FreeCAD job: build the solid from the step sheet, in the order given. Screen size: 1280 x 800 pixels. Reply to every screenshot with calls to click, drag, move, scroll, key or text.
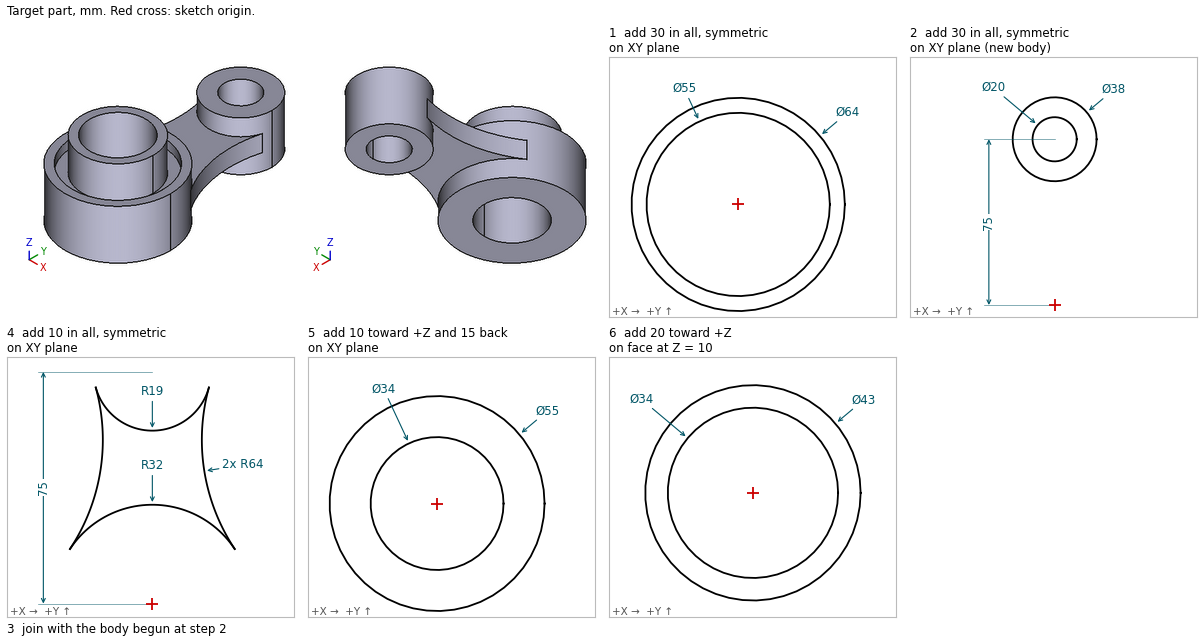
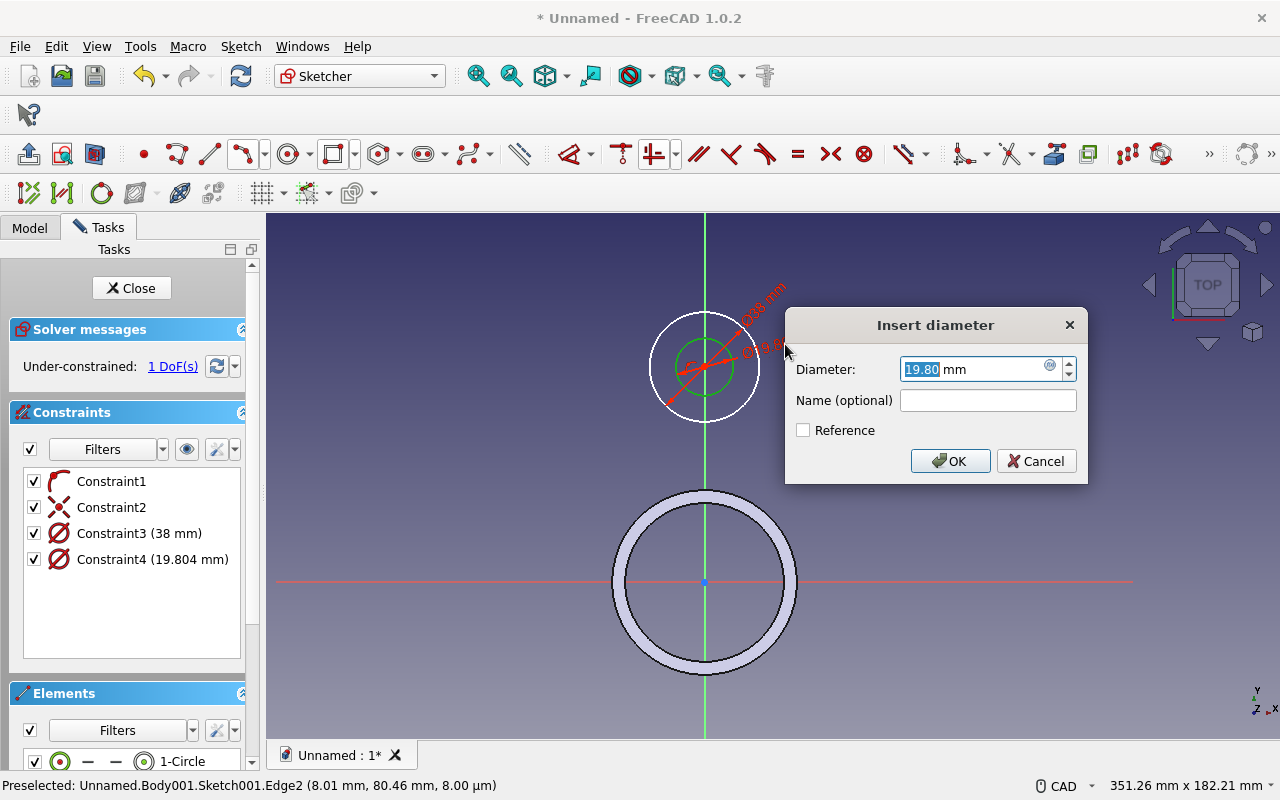
text(20)
key(Return)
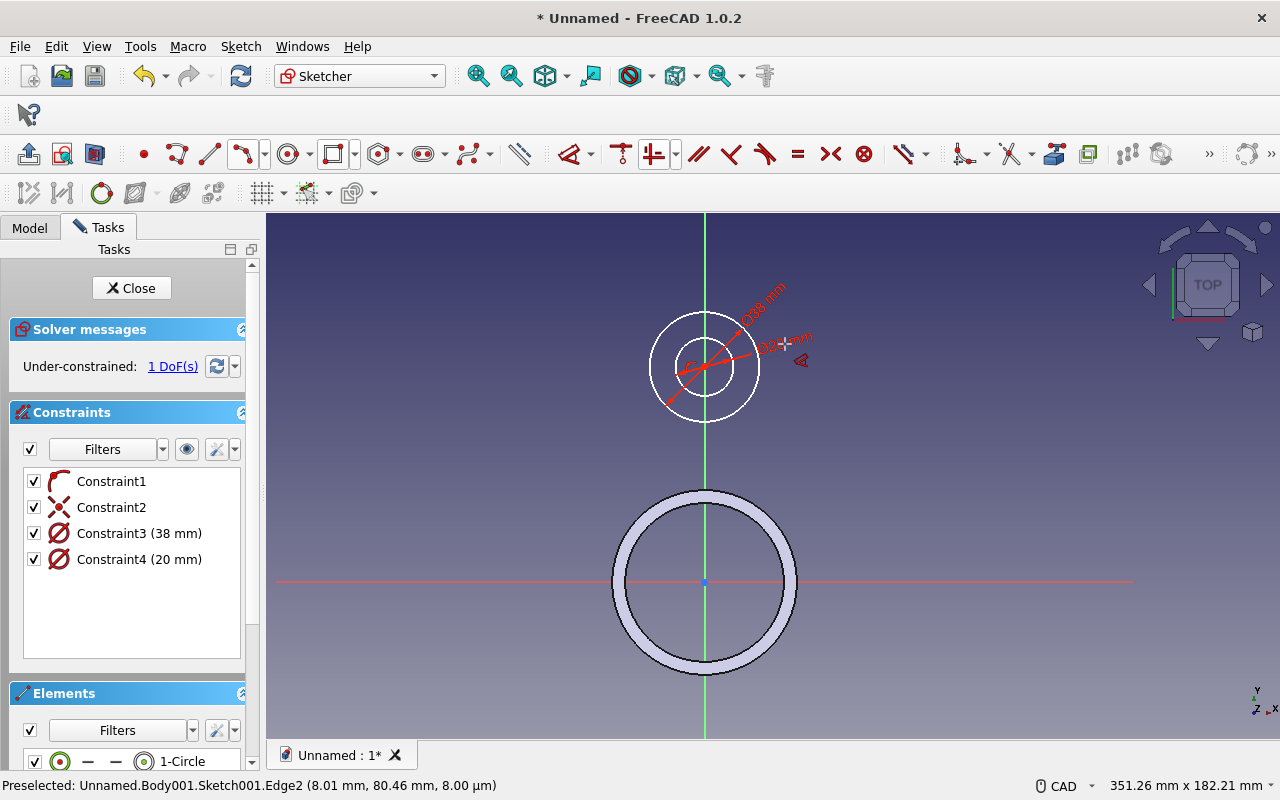
click(705, 367)
click(739, 475)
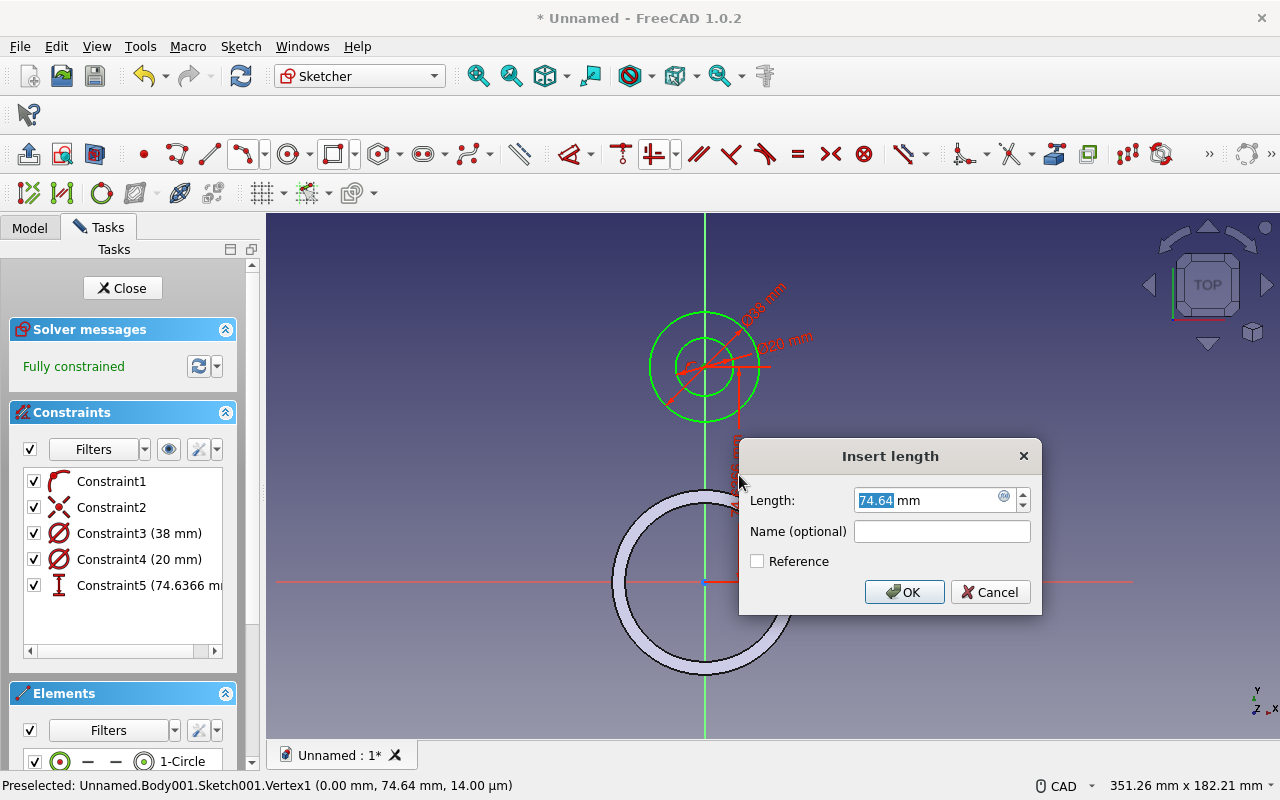
text(75)
key(Return)
key(Escape)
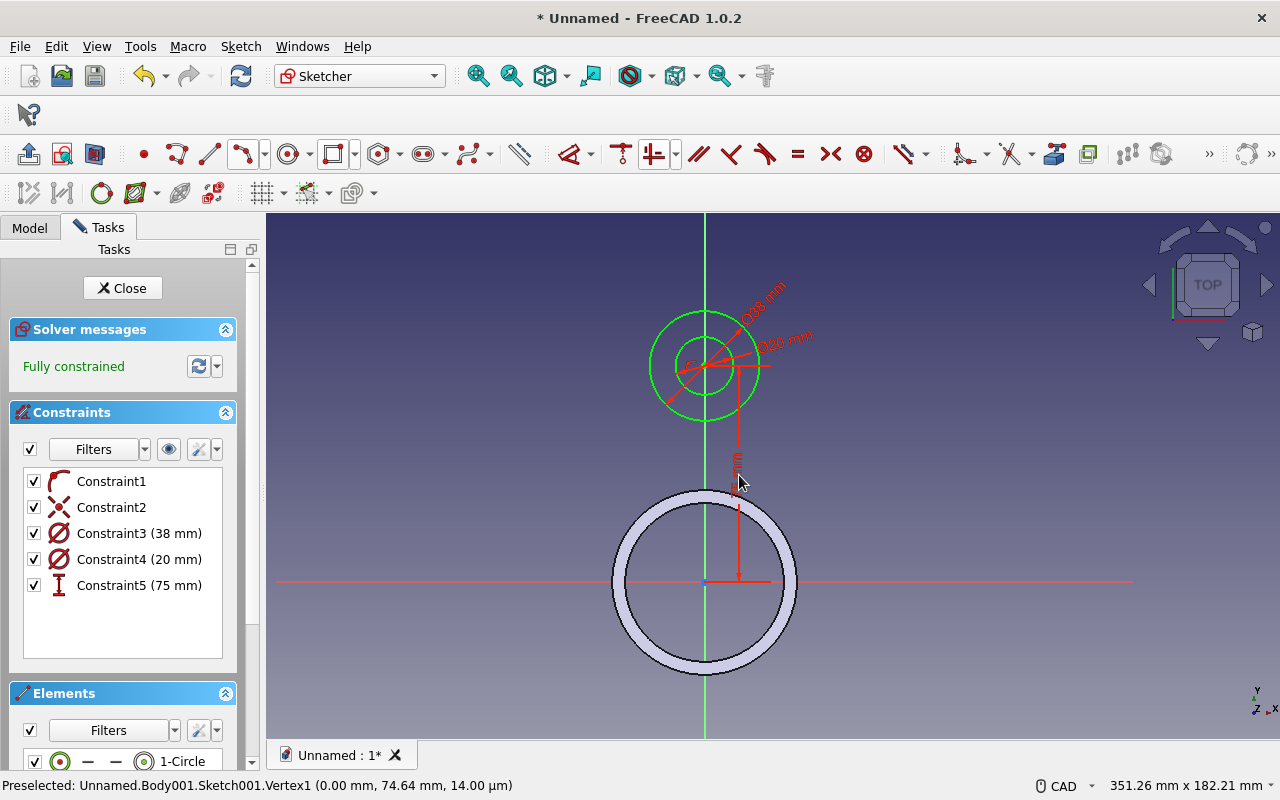
click(123, 288)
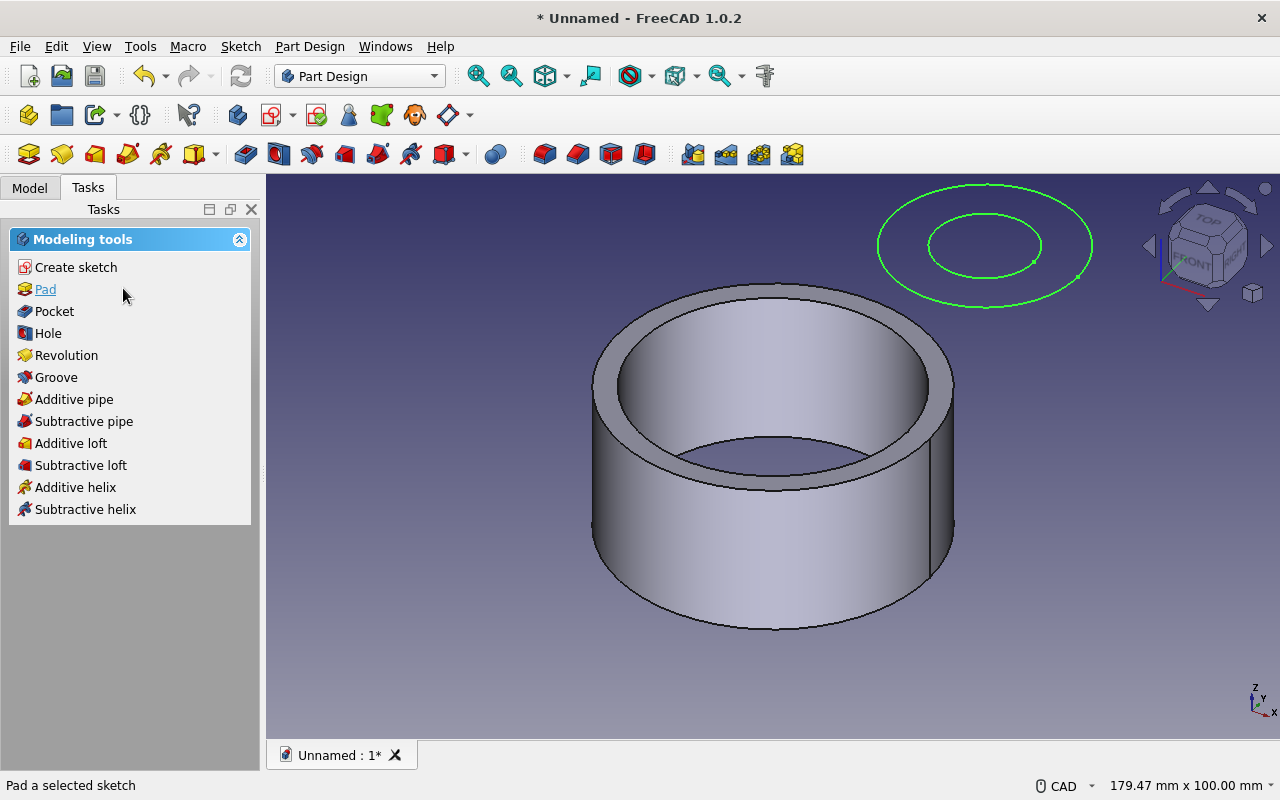
click(29, 154)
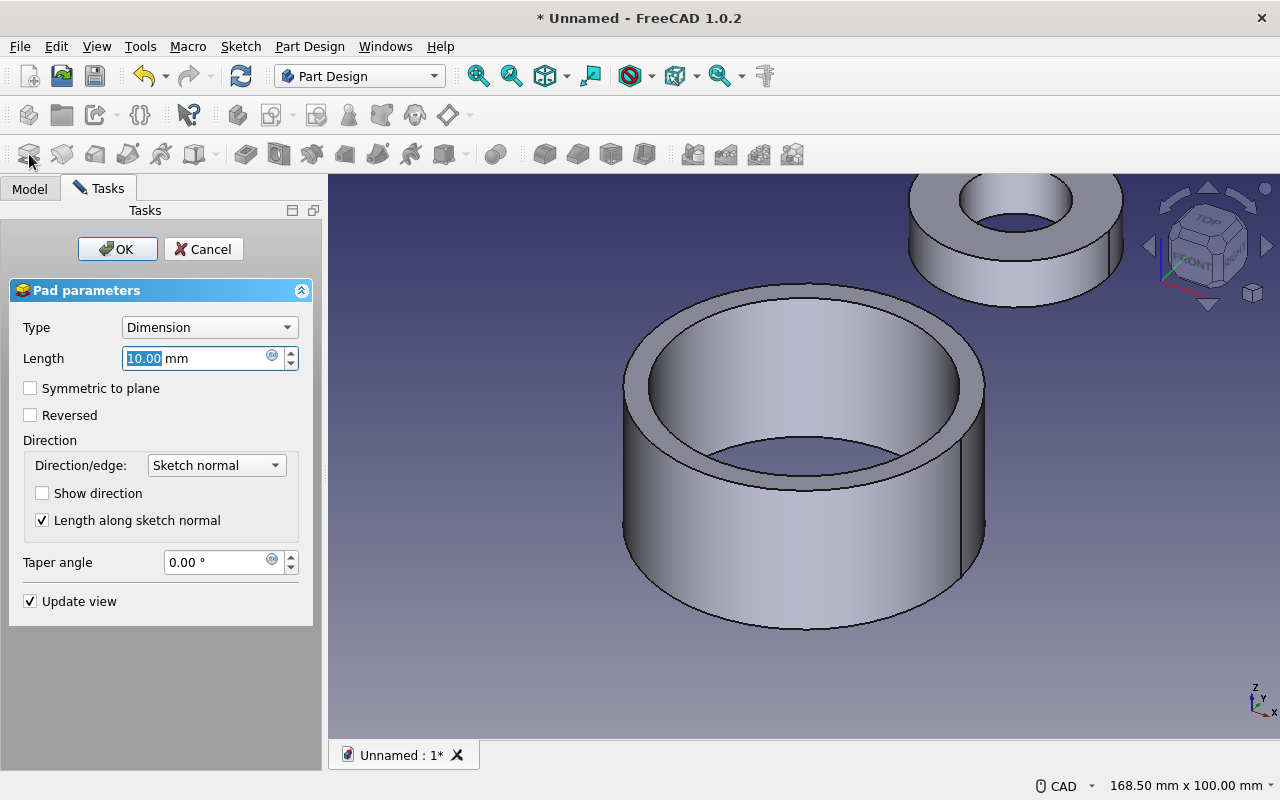
text(30)
key(Tab)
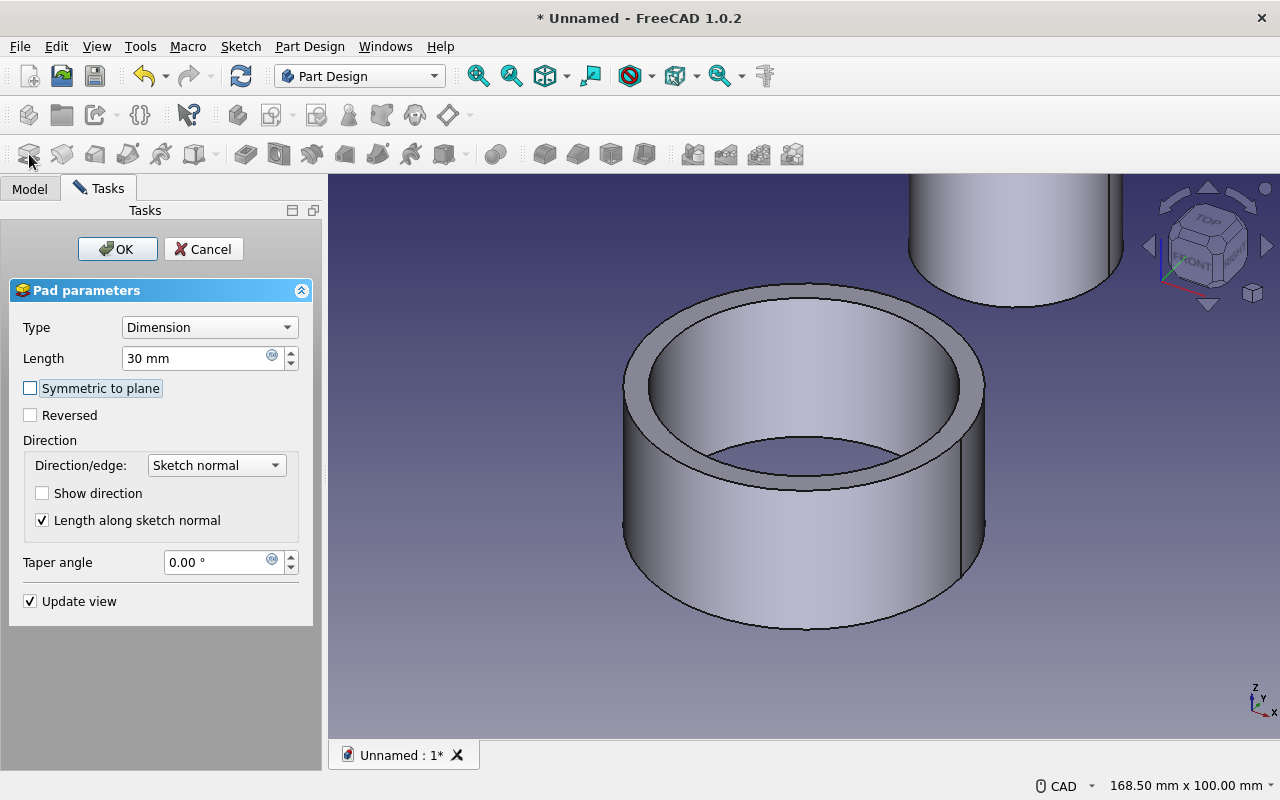
click(31, 388)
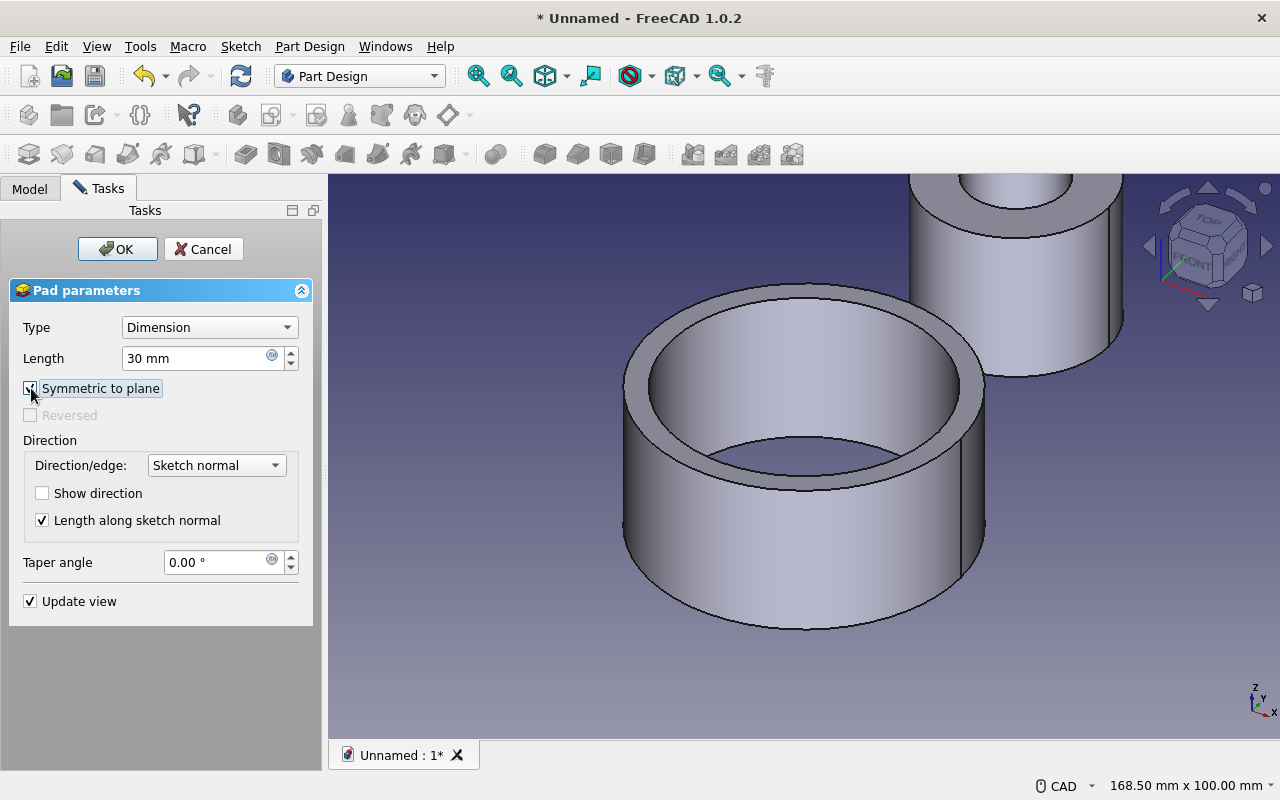
click(118, 249)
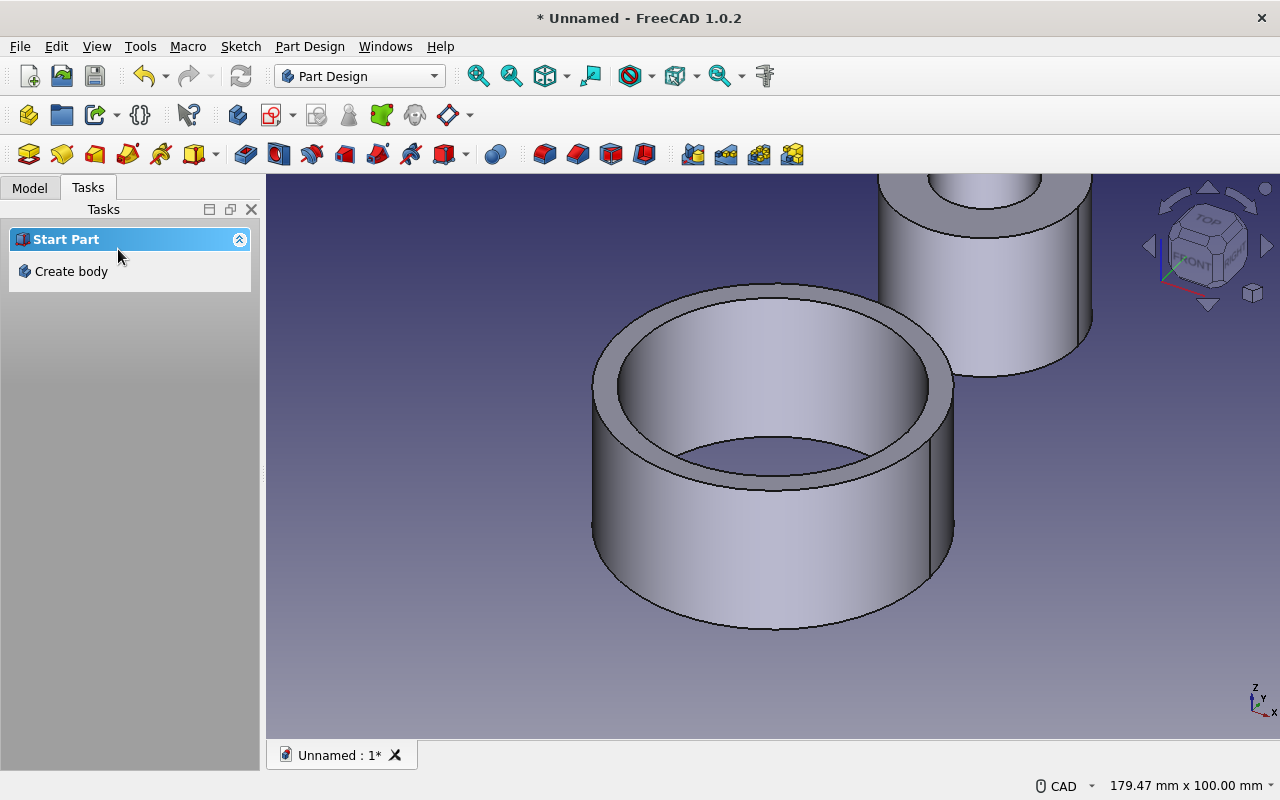
key(v)
key(f)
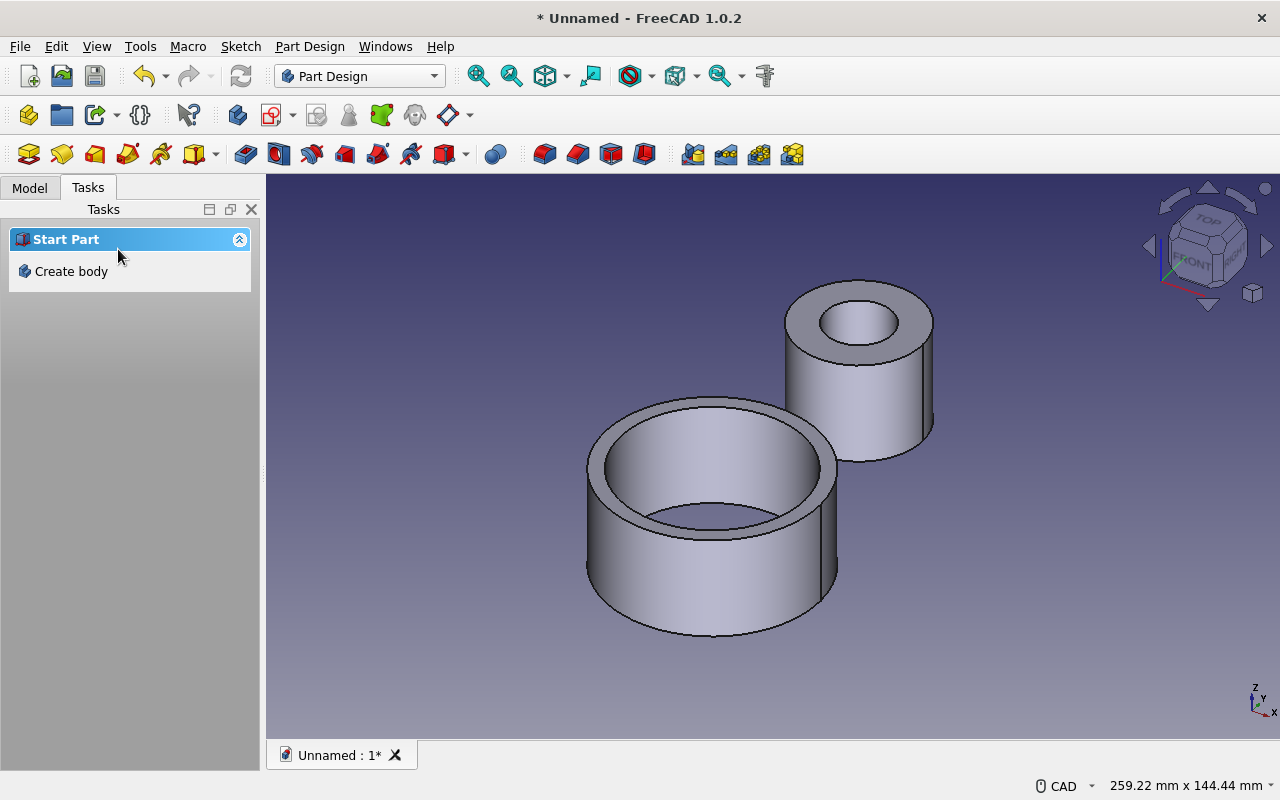
click(30, 188)